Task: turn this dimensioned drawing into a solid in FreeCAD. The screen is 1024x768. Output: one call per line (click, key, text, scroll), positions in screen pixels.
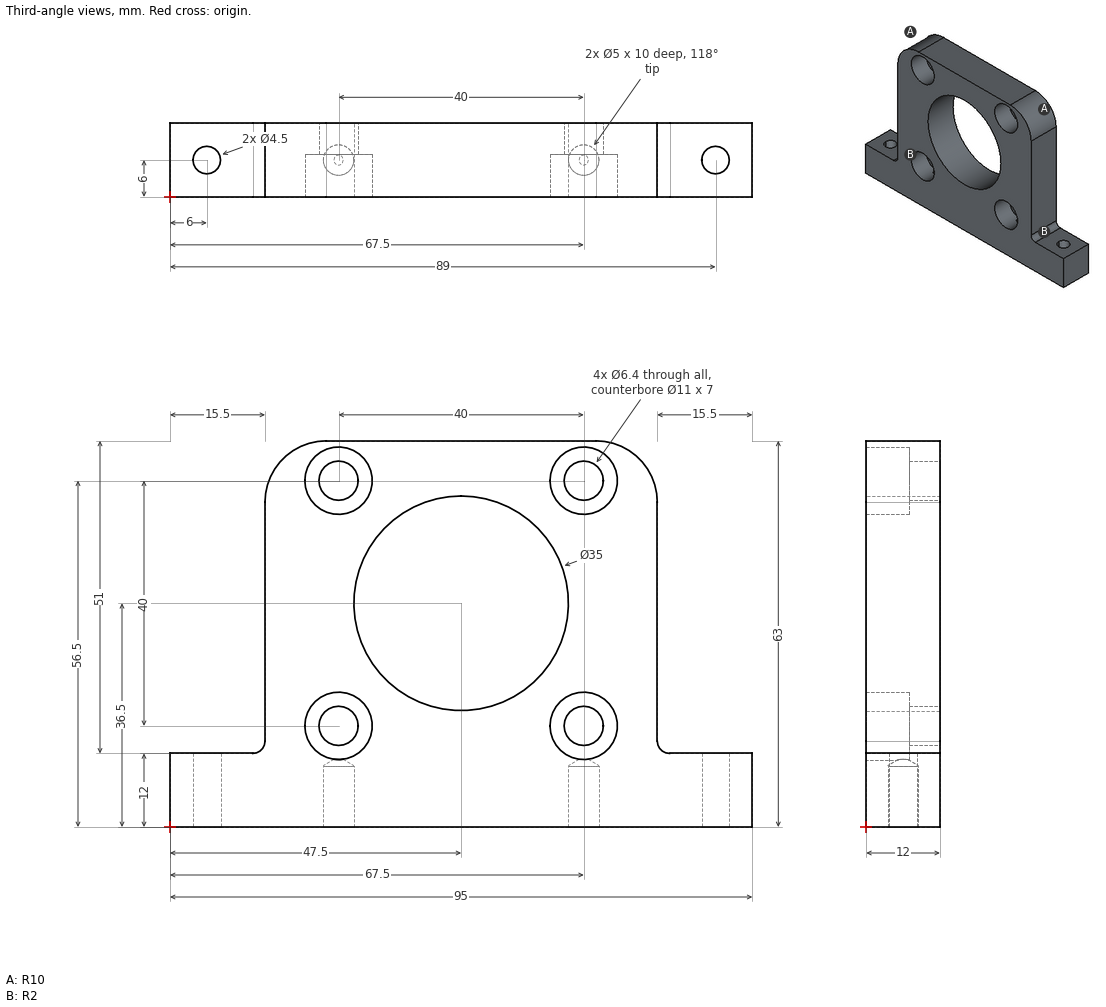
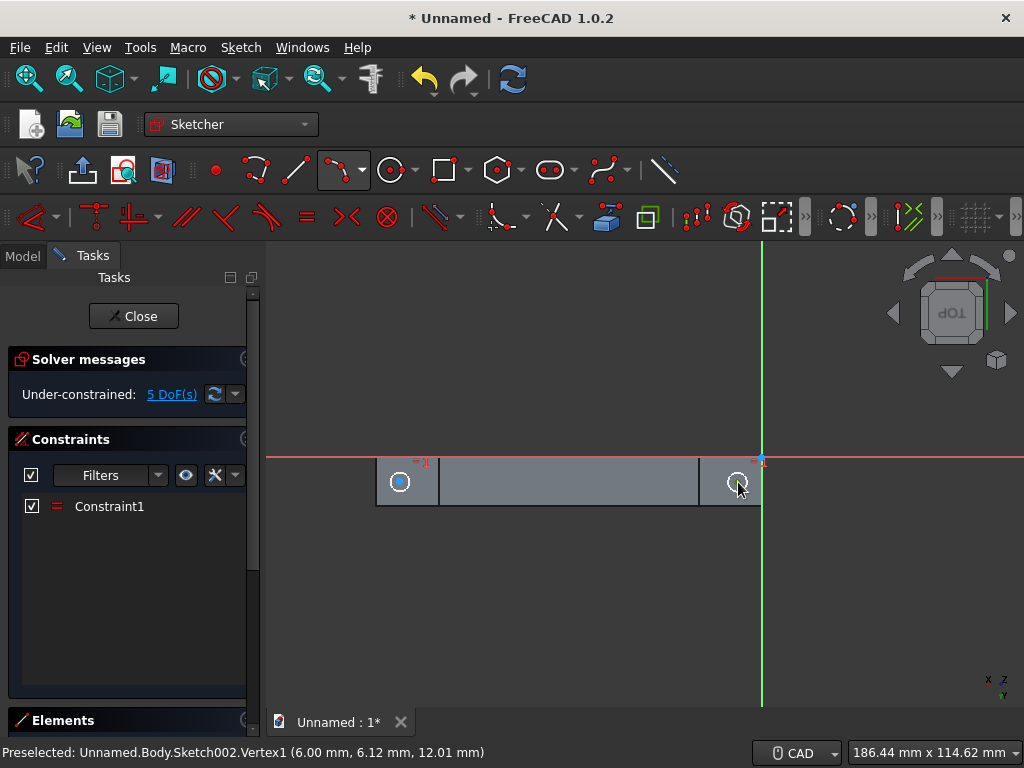
click(400, 482)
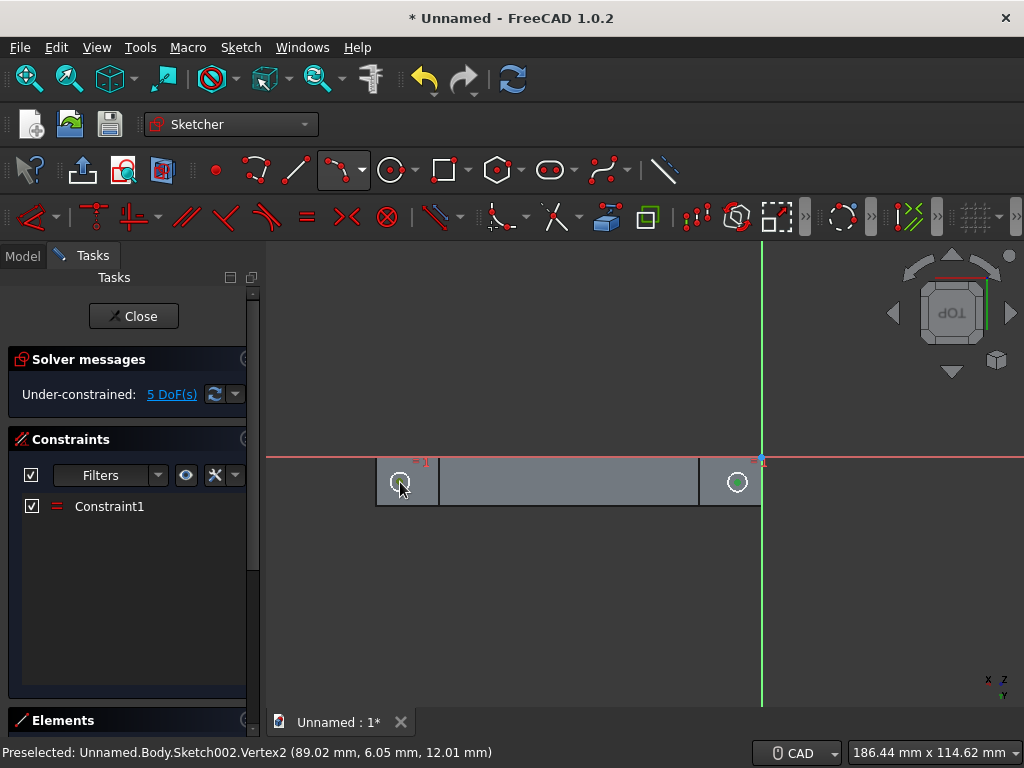
click(160, 218)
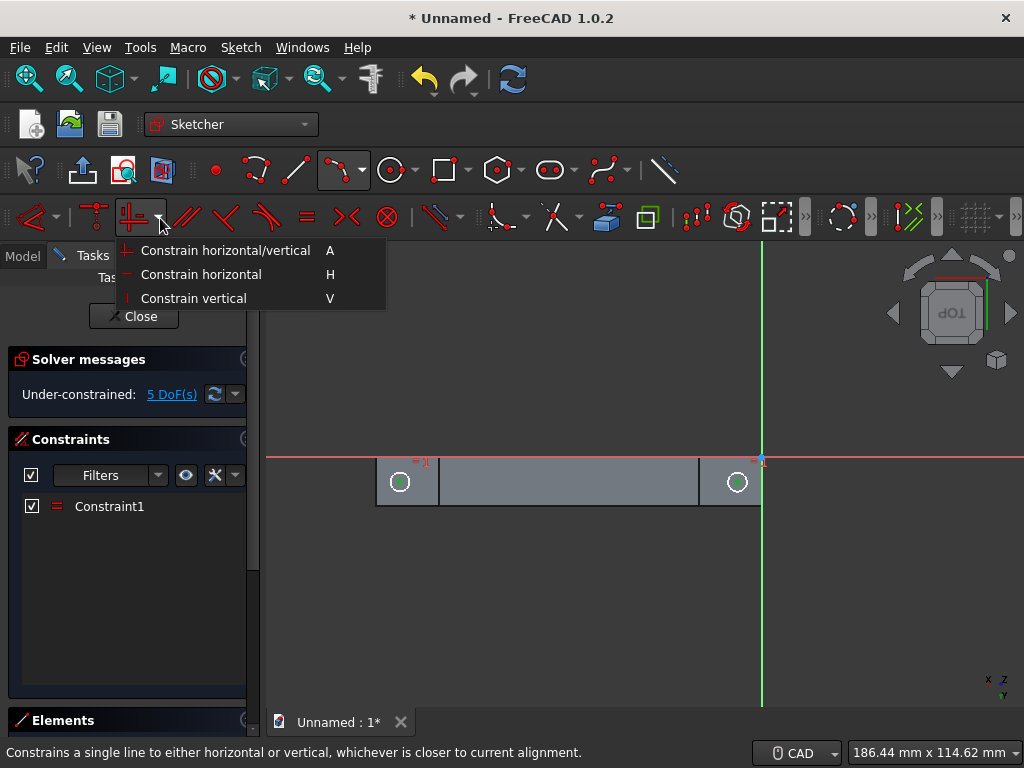
click(251, 274)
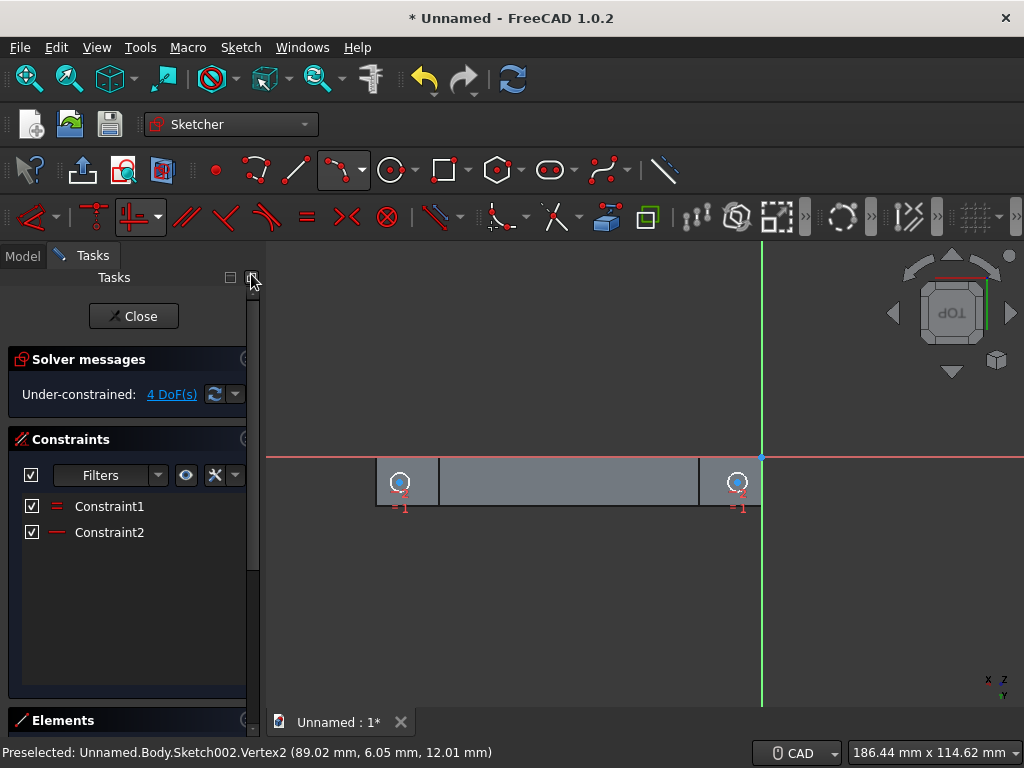
click(32, 218)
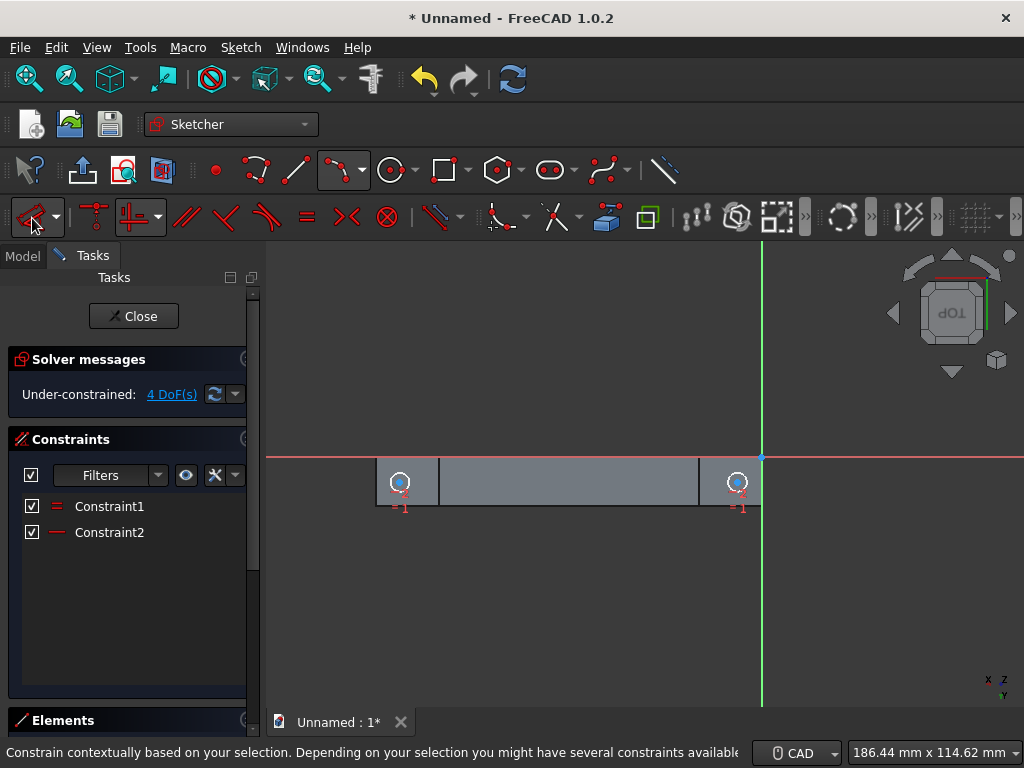
scroll(744, 476, up, 4)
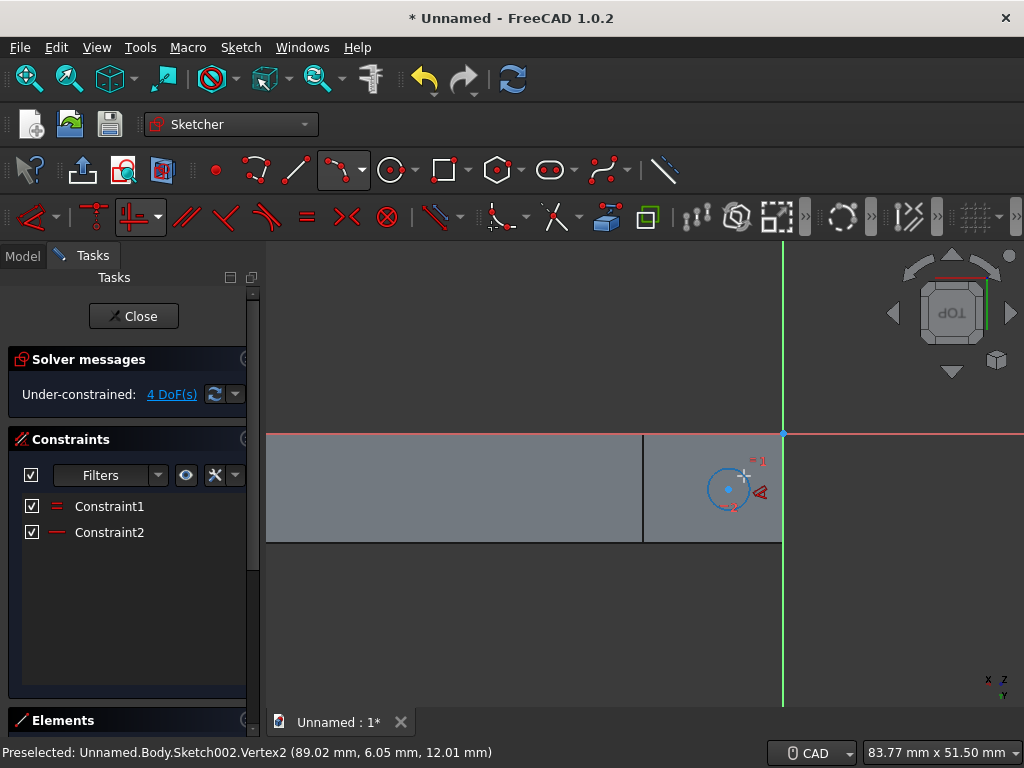
click(743, 475)
click(766, 452)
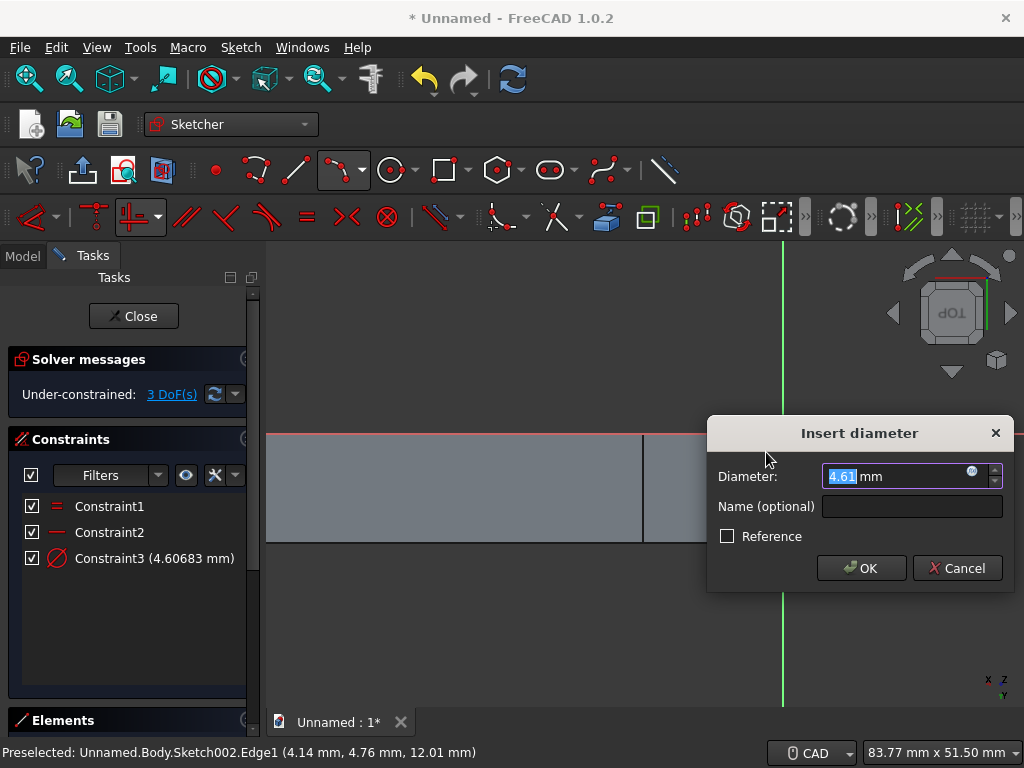
text(4.5)
key(Return)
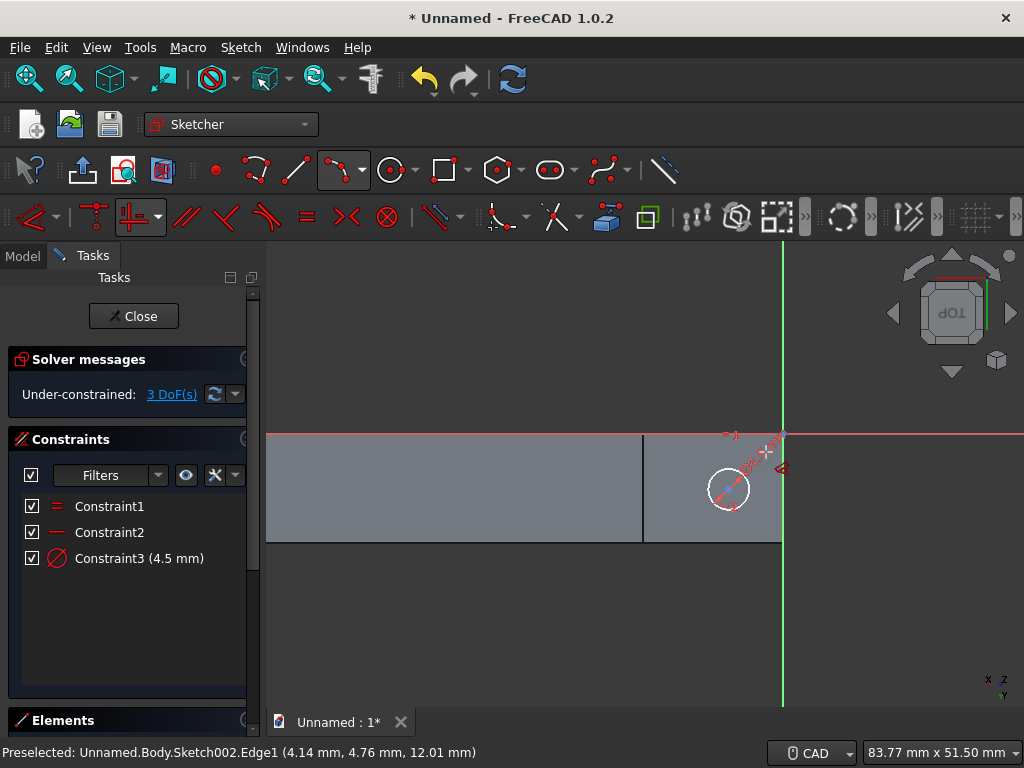
click(729, 489)
click(756, 400)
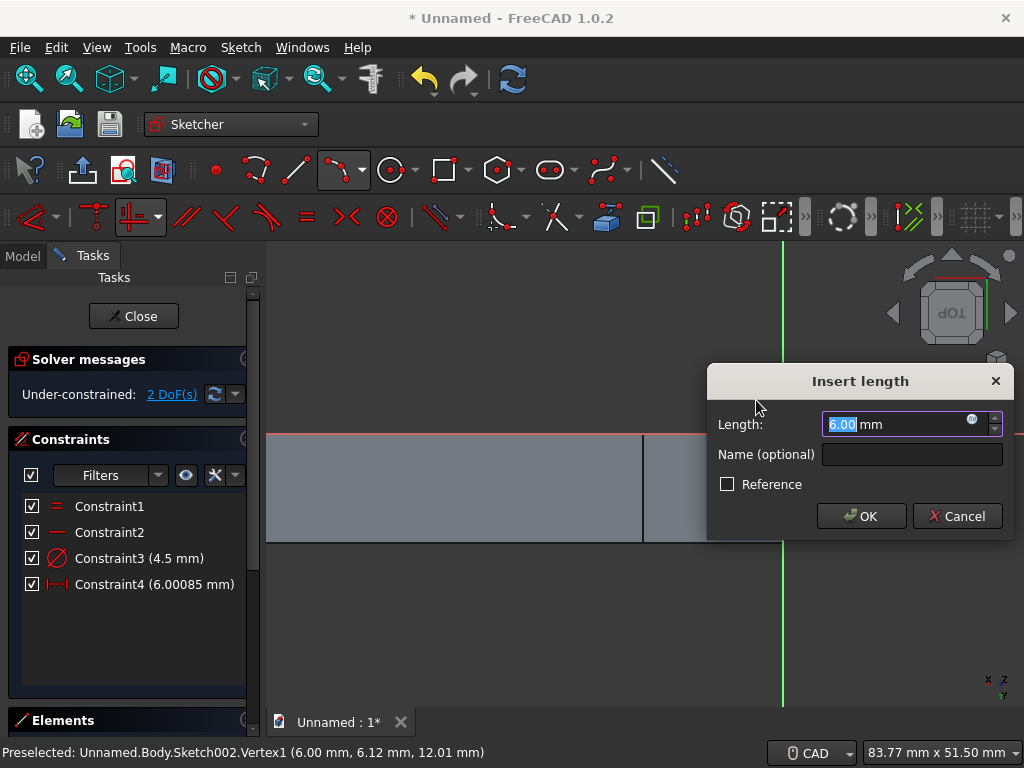
text(6)
key(Return)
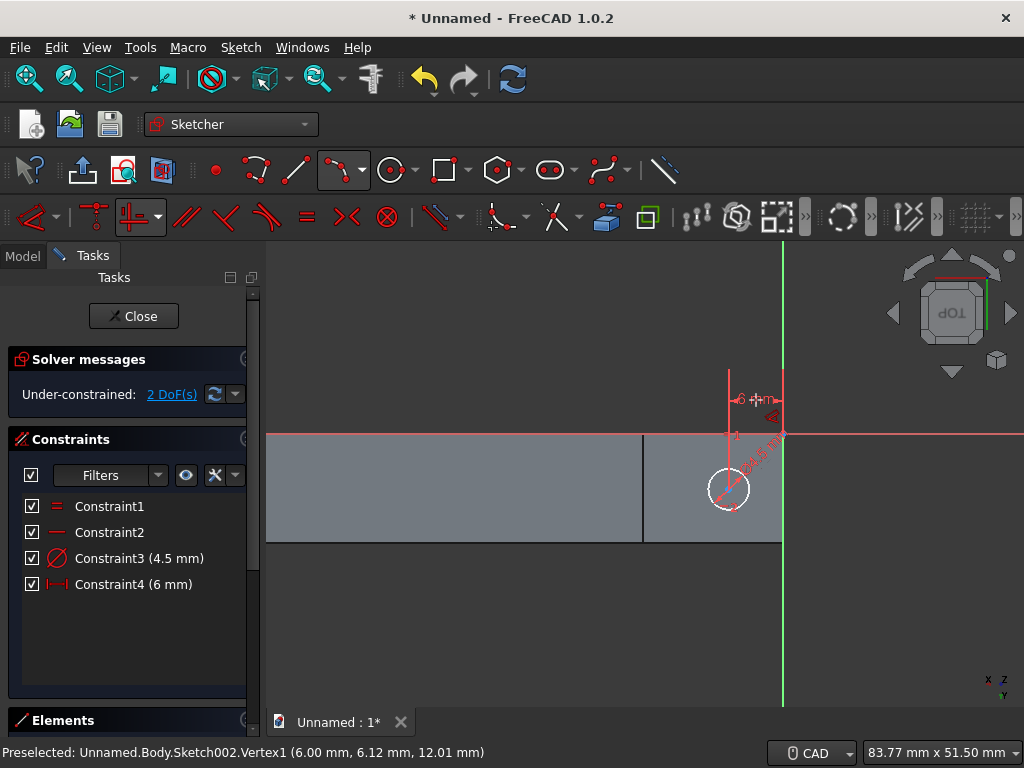
click(729, 489)
click(817, 474)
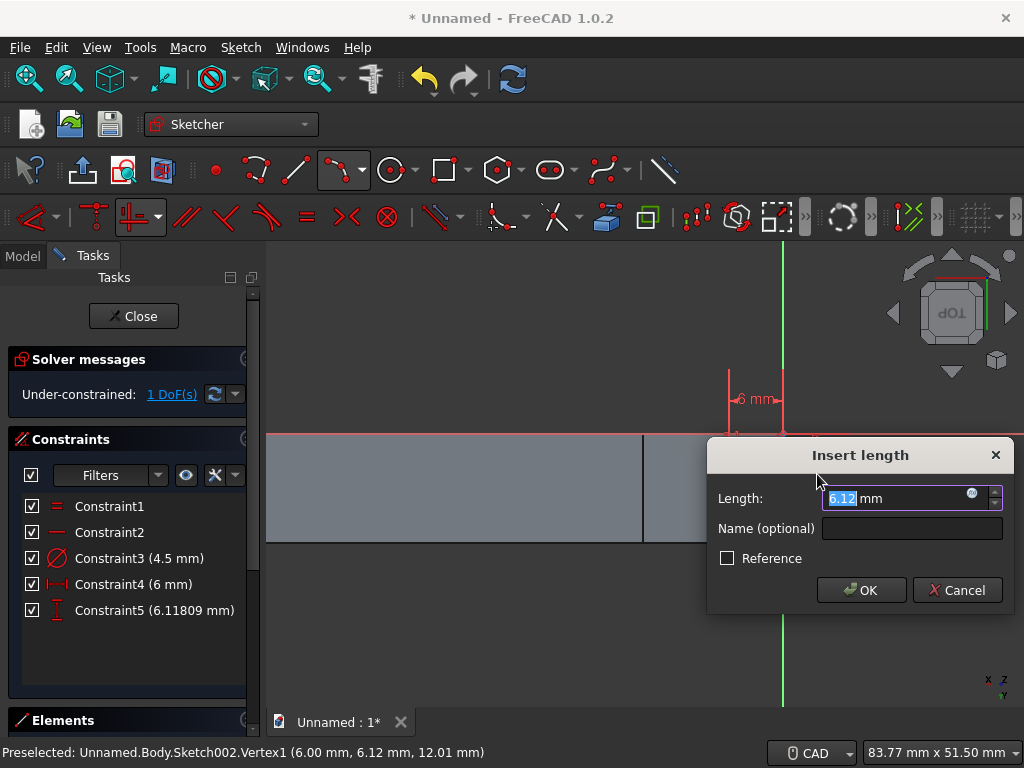
text(6)
key(Return)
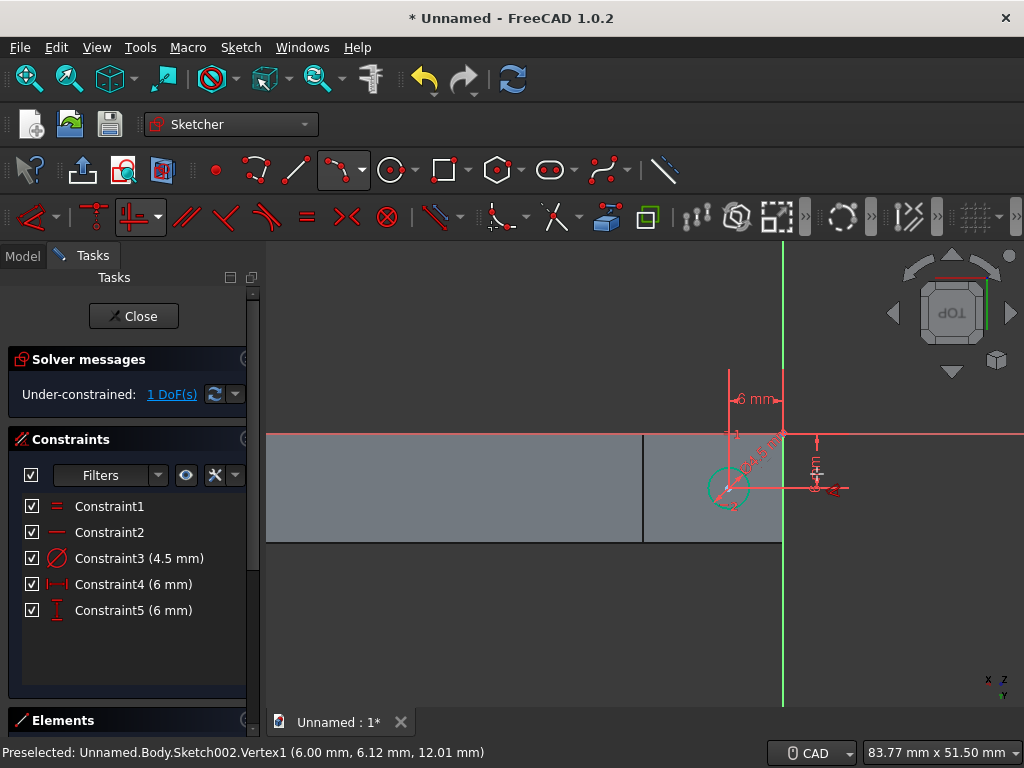
scroll(745, 476, down, 4)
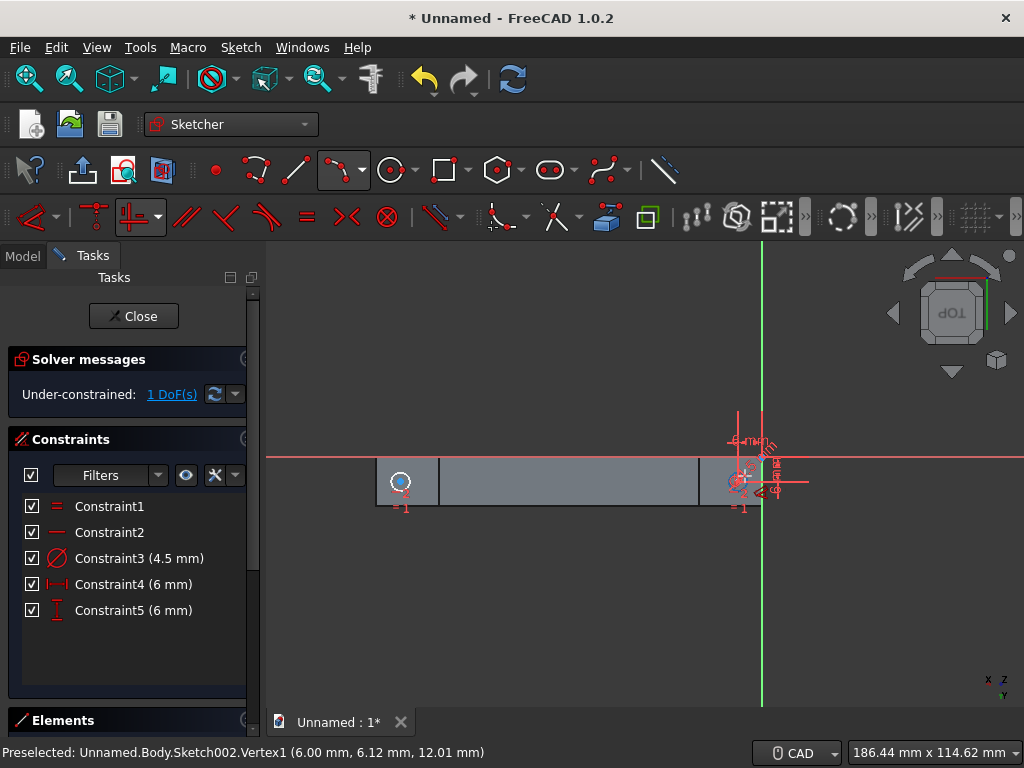
click(401, 482)
click(581, 423)